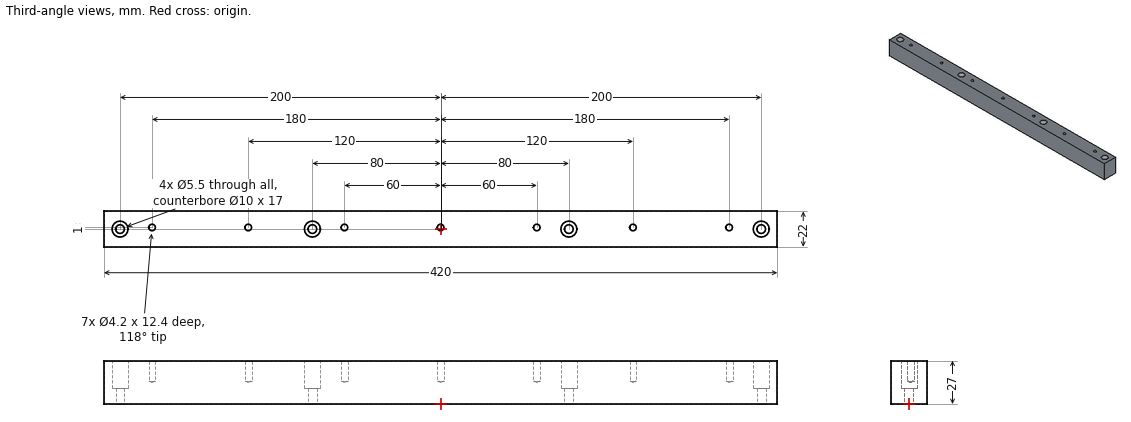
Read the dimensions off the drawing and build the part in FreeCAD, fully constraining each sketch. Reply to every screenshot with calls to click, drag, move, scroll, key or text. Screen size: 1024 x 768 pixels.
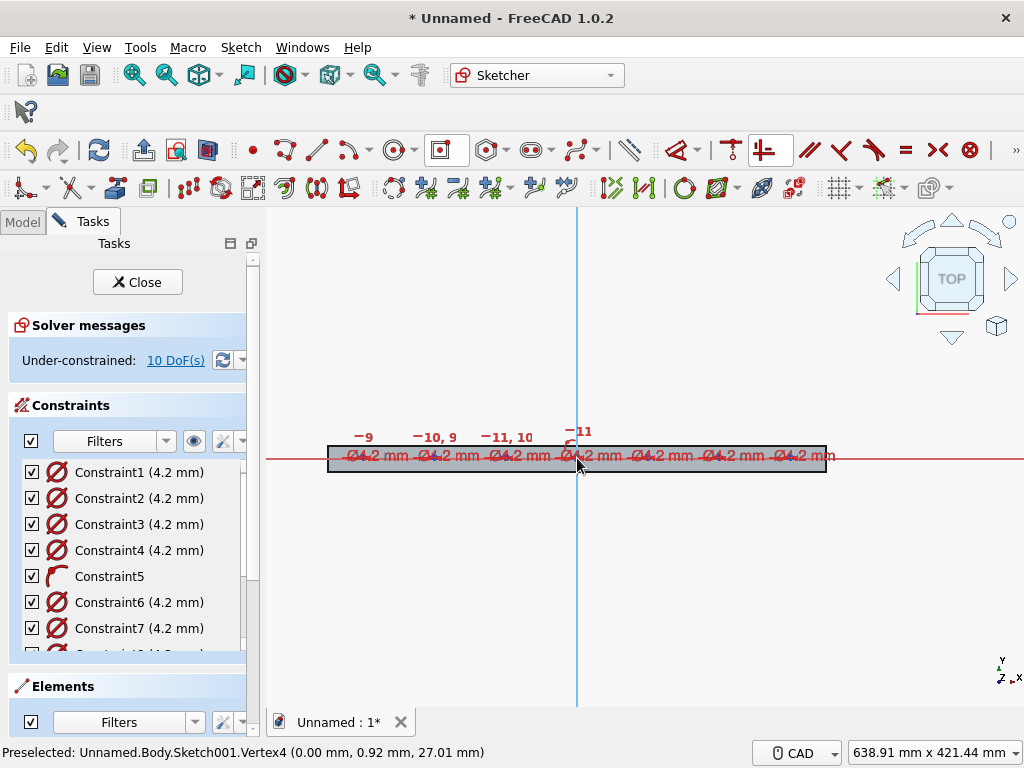
click(648, 458)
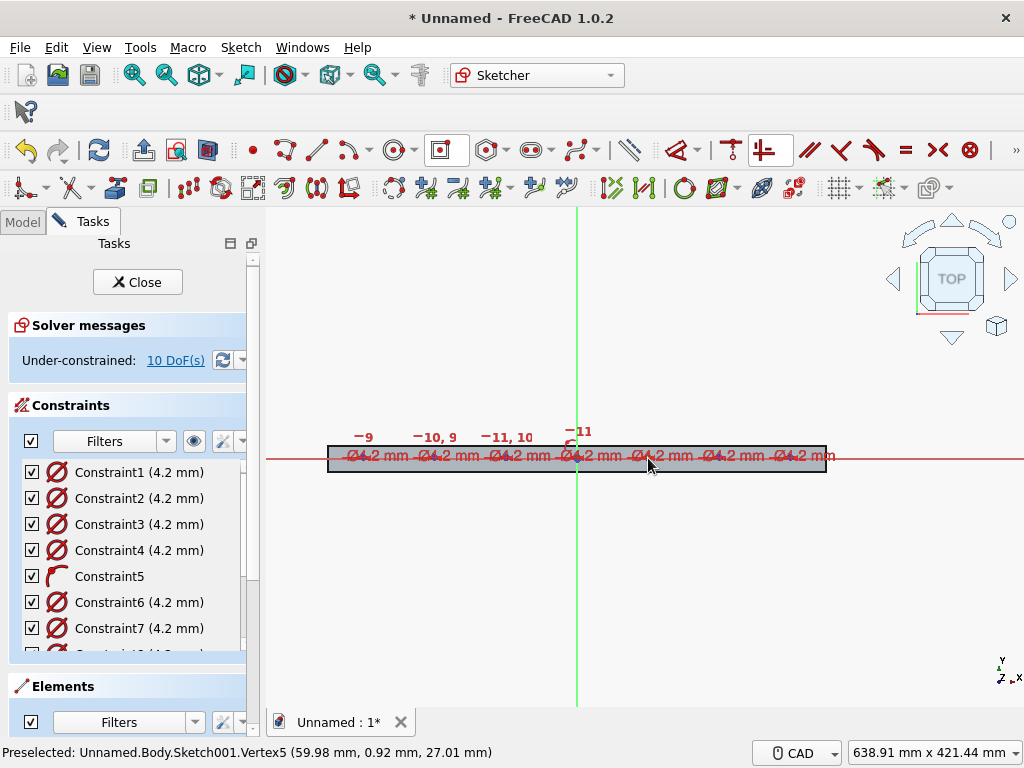
key(h)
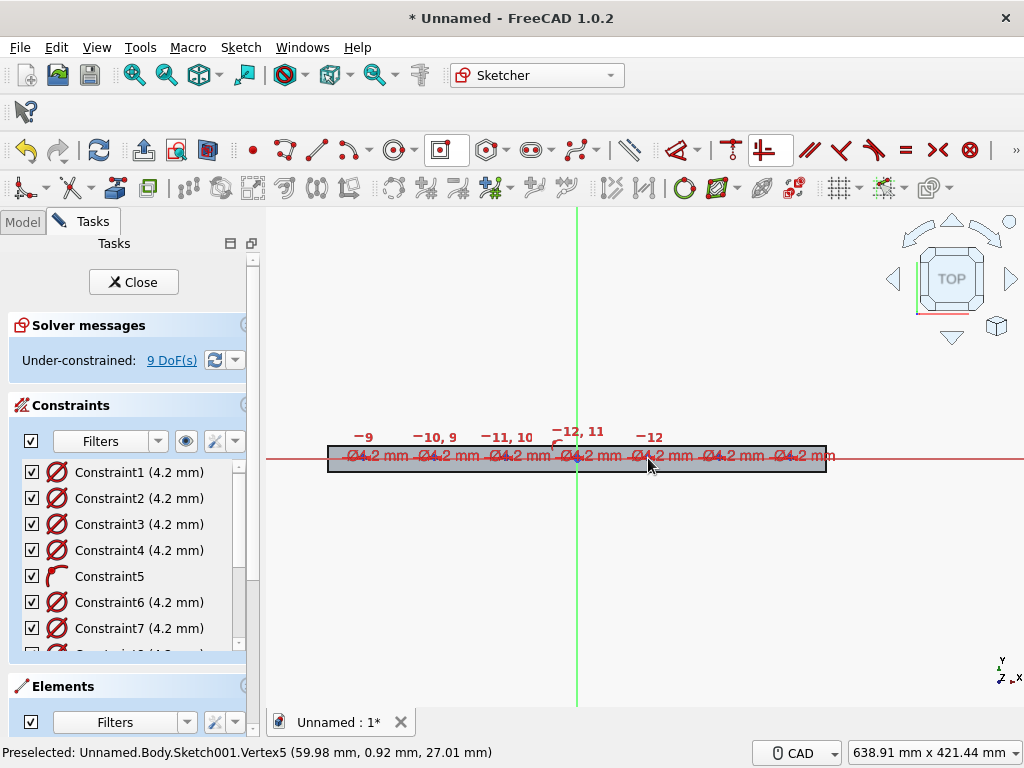
click(648, 458)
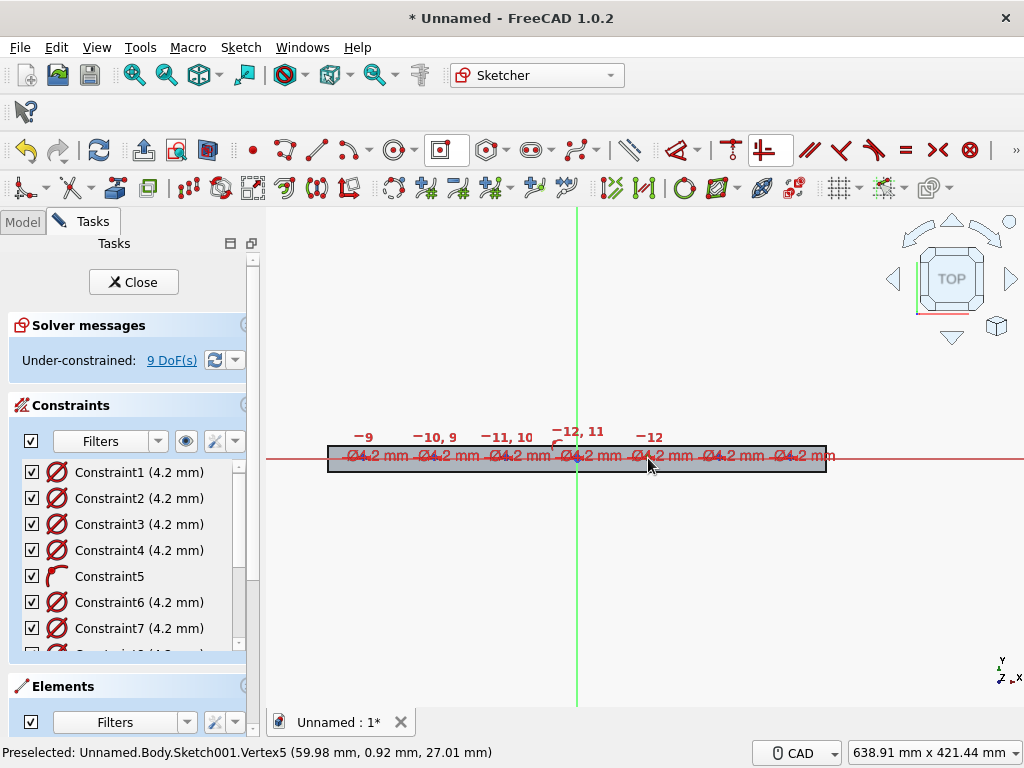
click(720, 458)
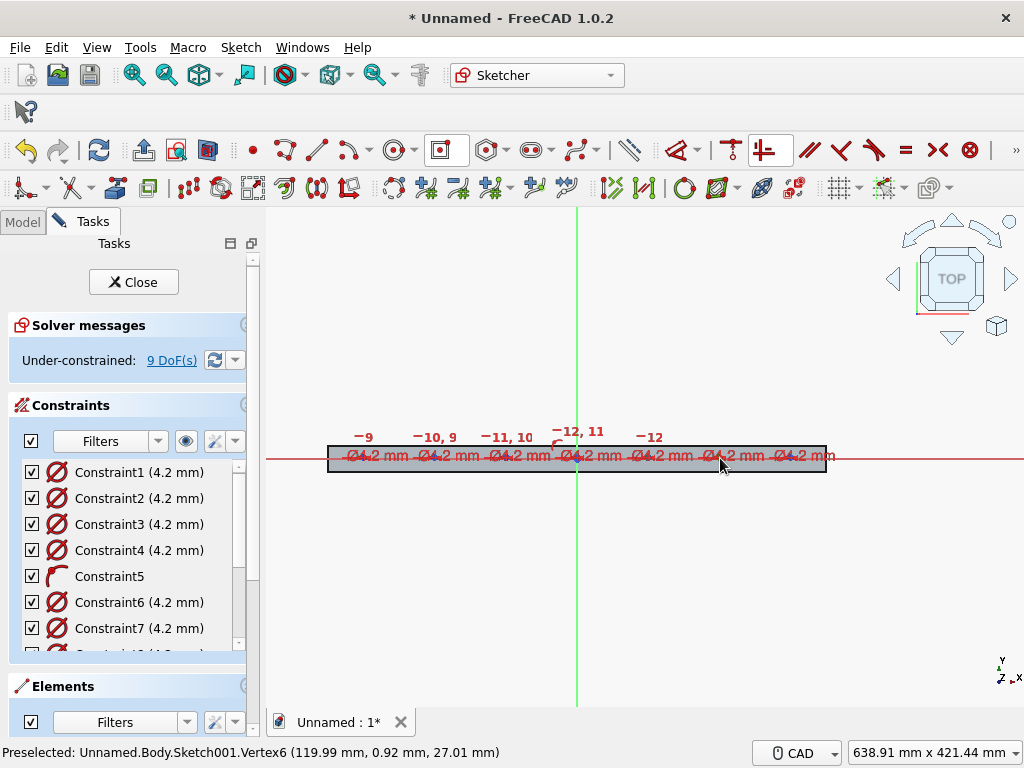
click(788, 150)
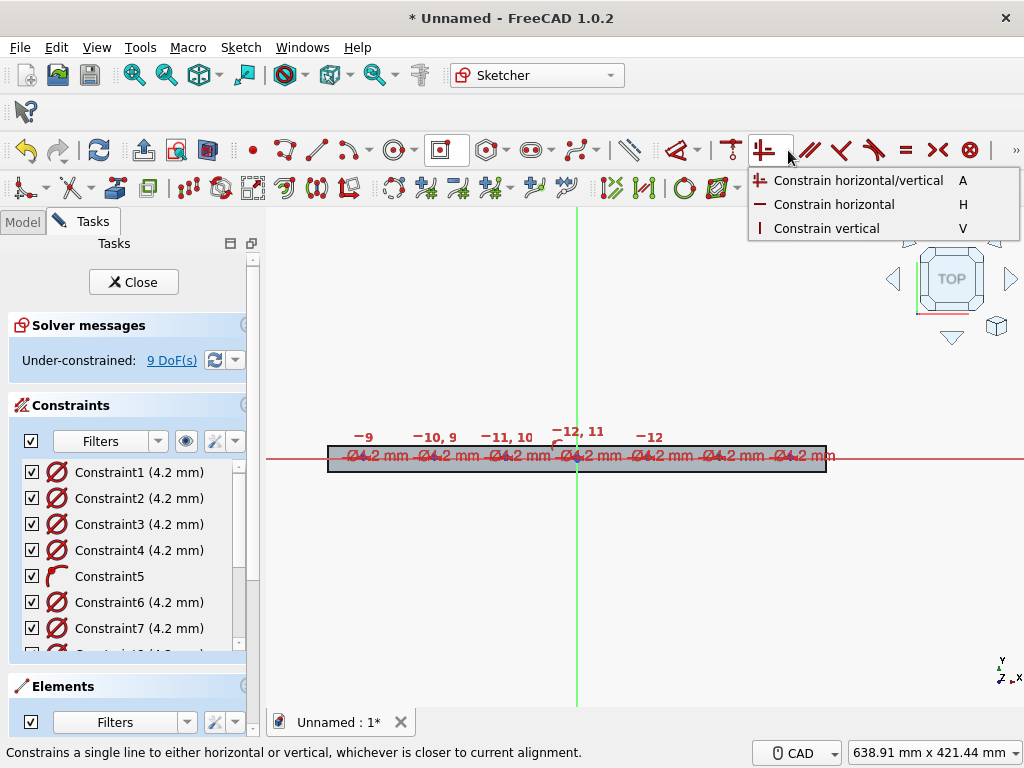
click(884, 204)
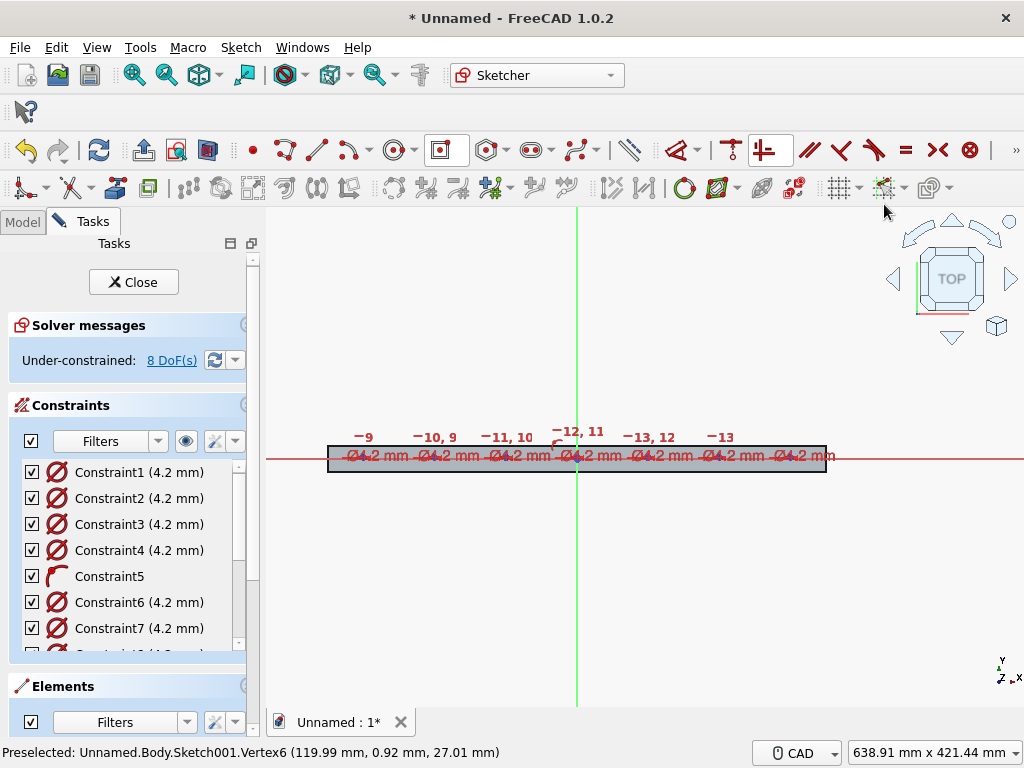
click(720, 458)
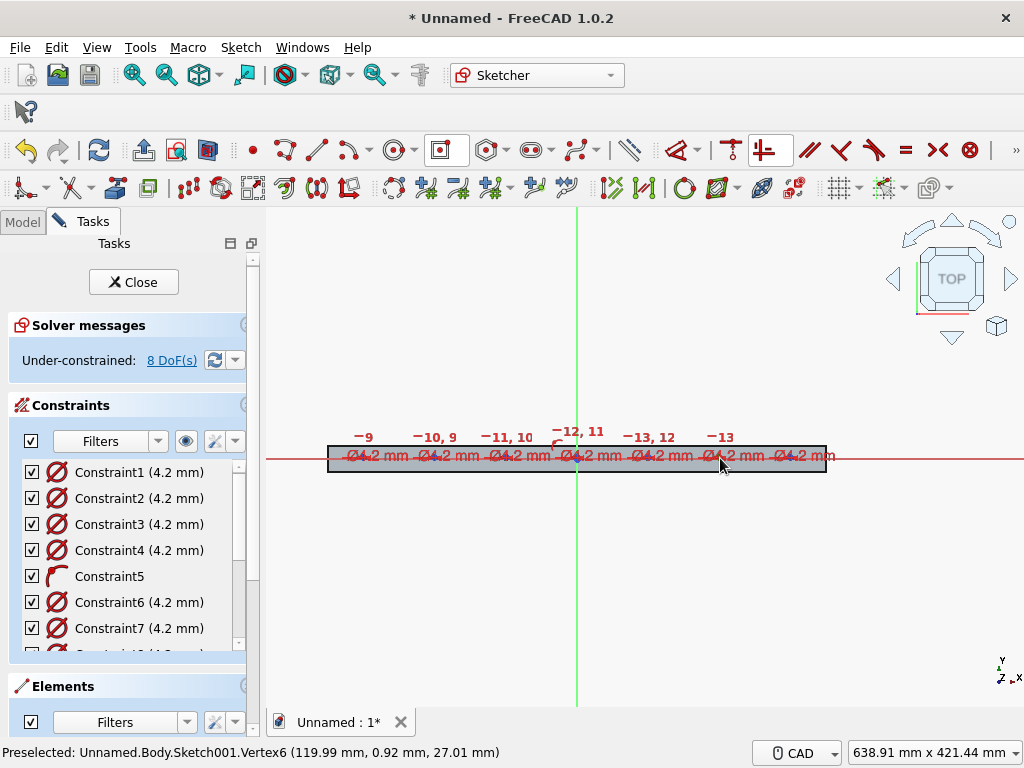
click(791, 458)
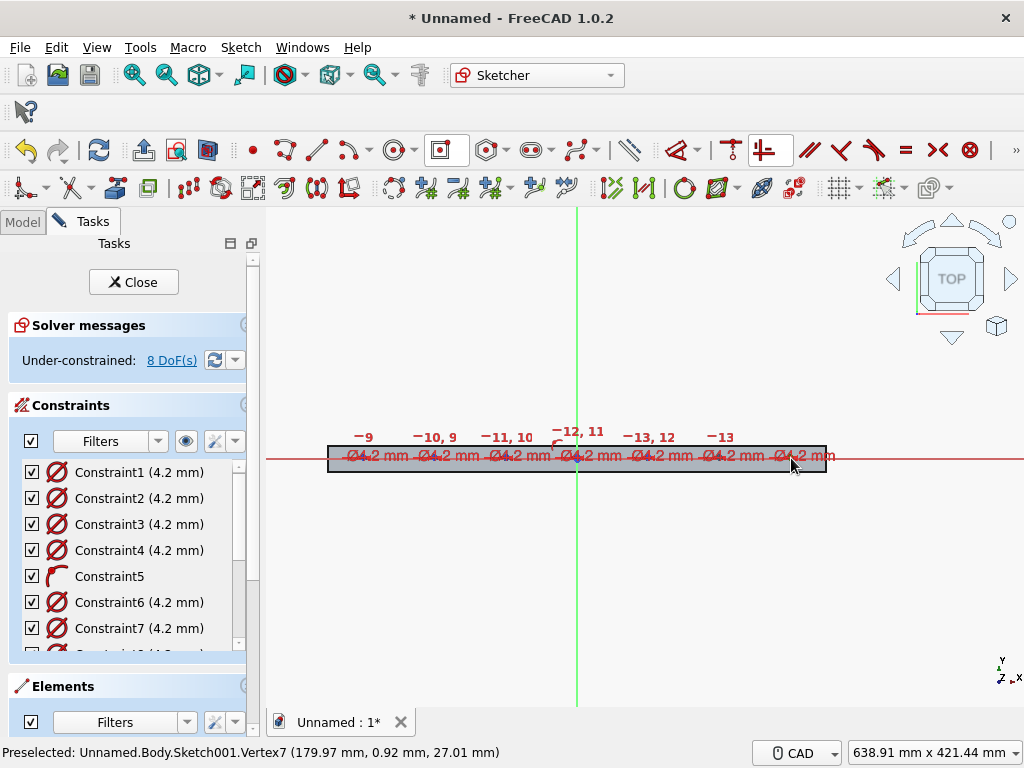
key(h)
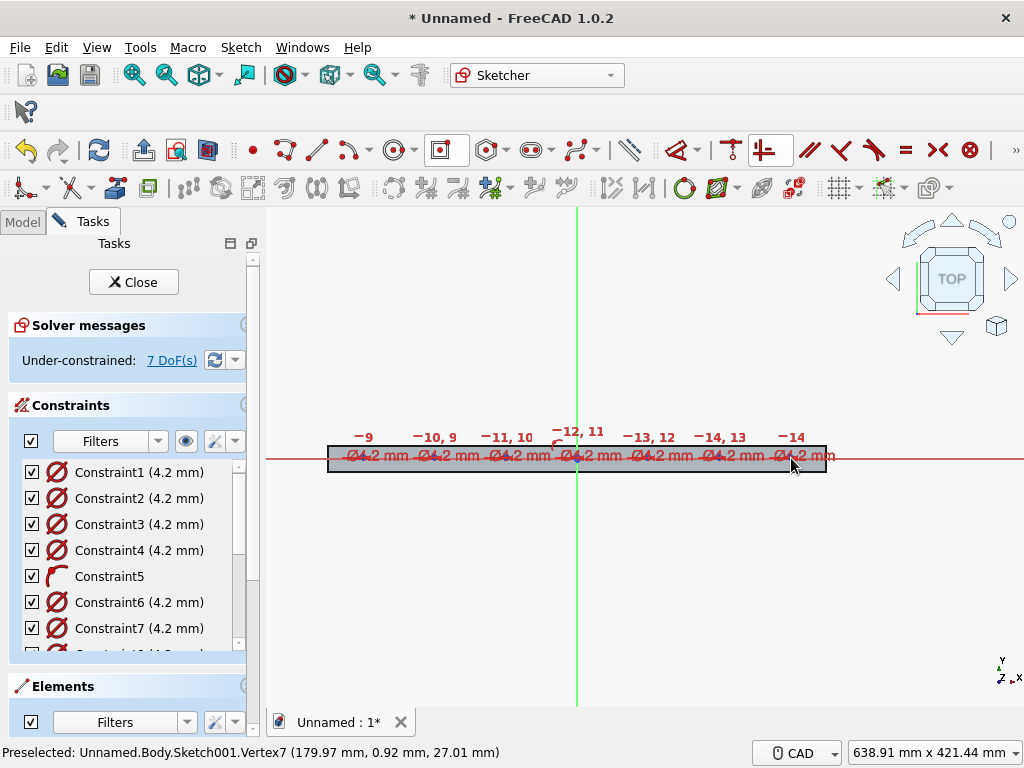
key(d)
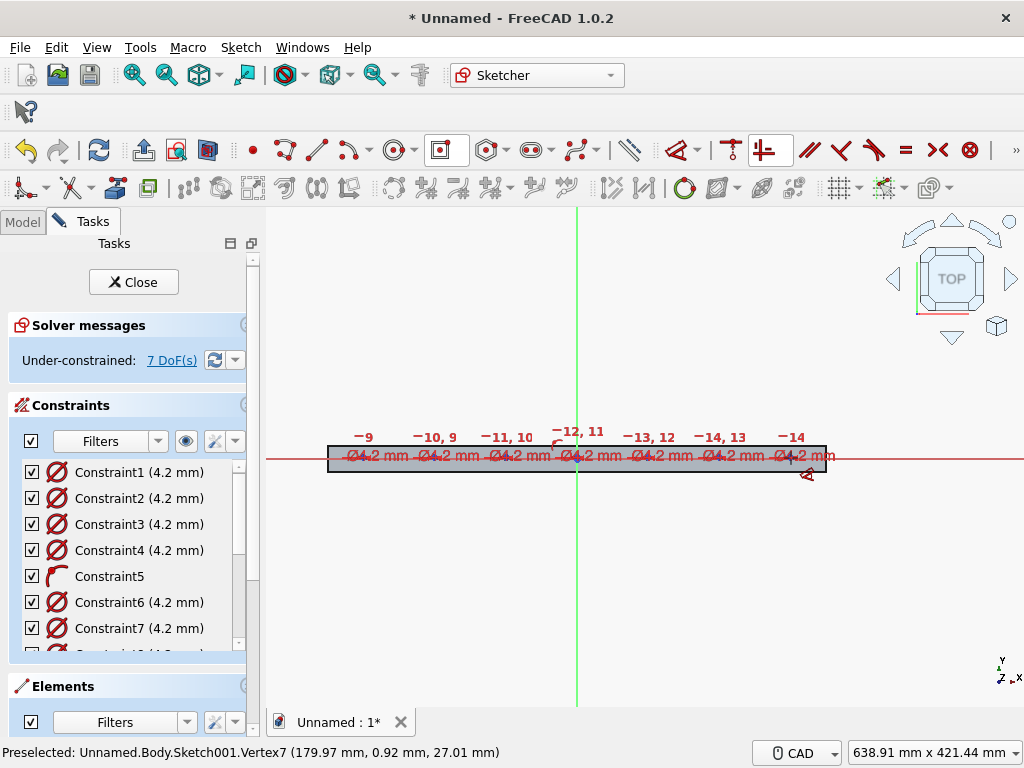
scroll(364, 458, up, 18)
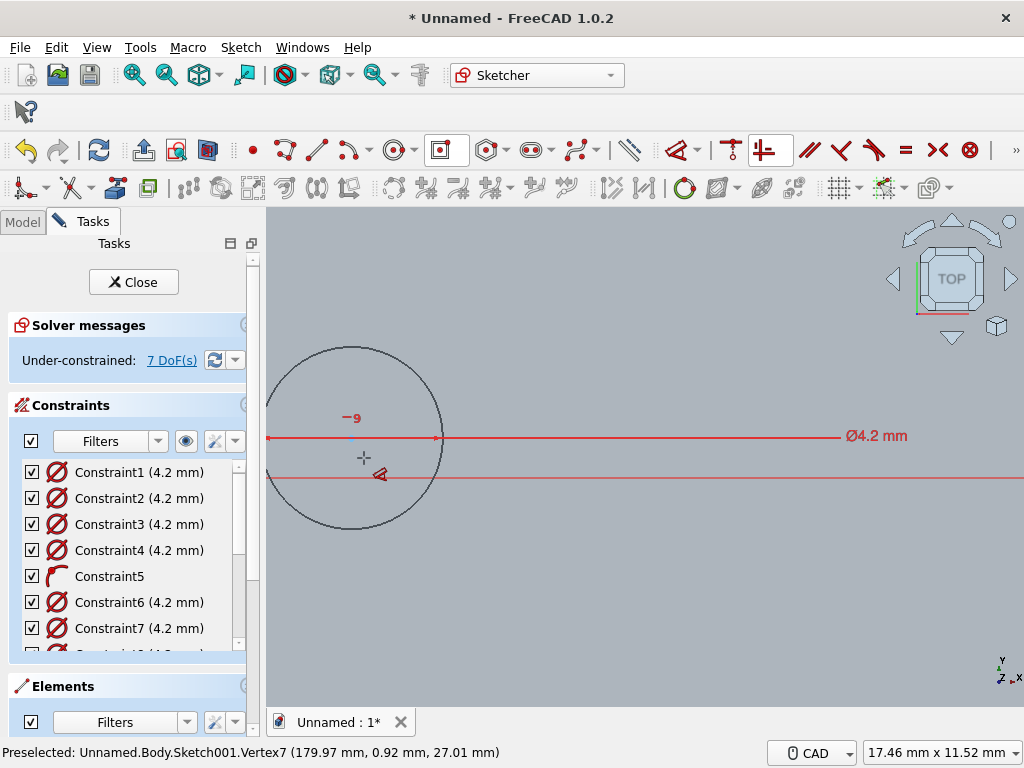
click(352, 438)
click(318, 458)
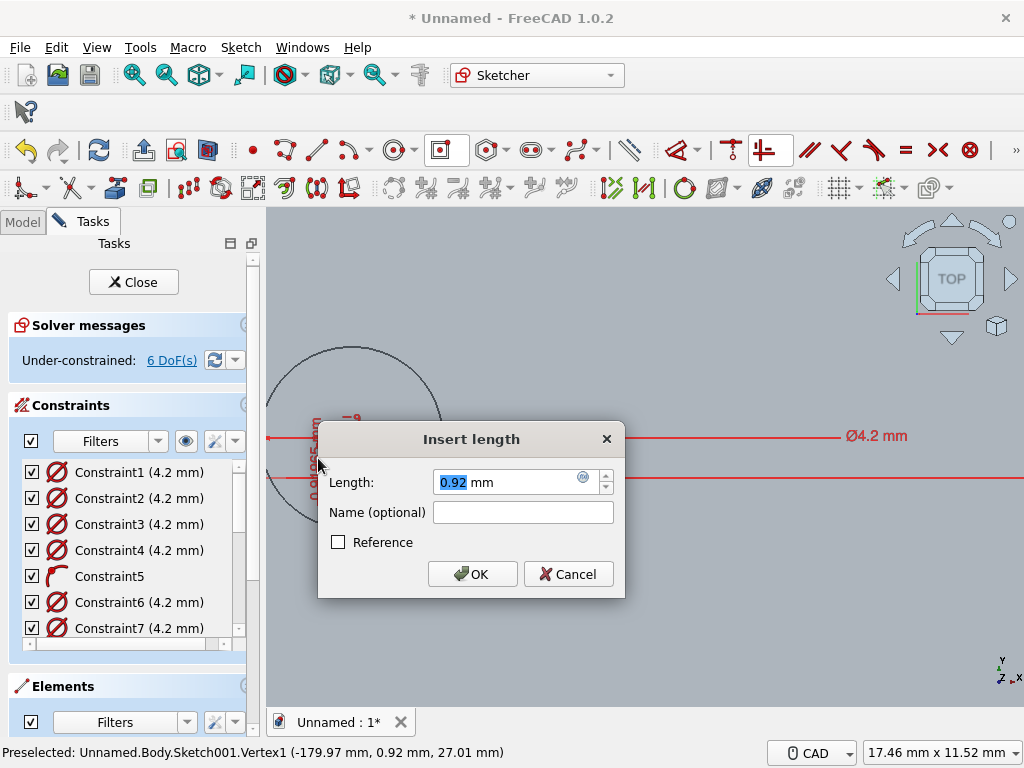
text(1)
key(Return)